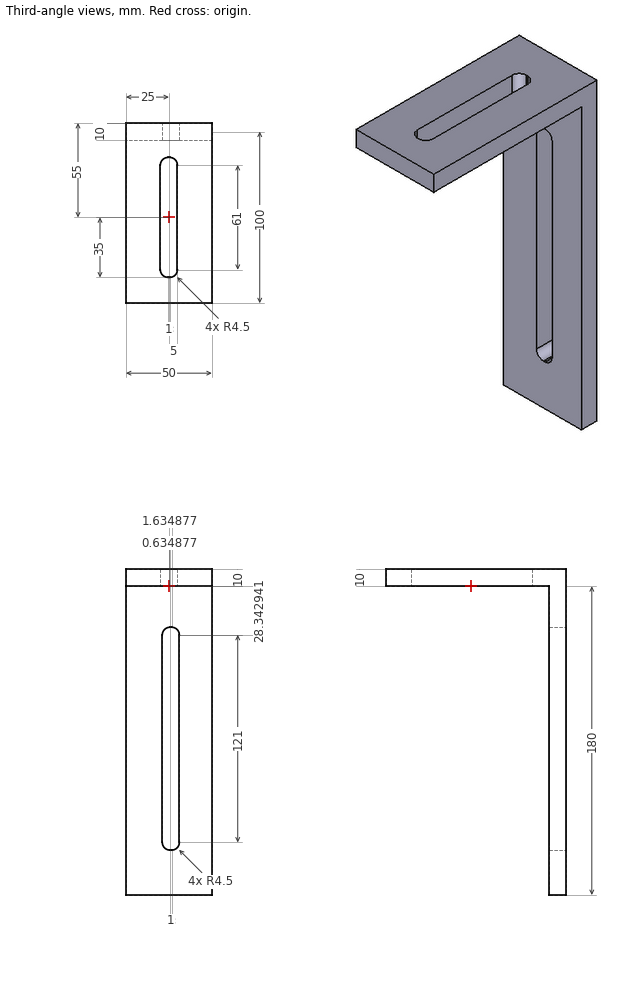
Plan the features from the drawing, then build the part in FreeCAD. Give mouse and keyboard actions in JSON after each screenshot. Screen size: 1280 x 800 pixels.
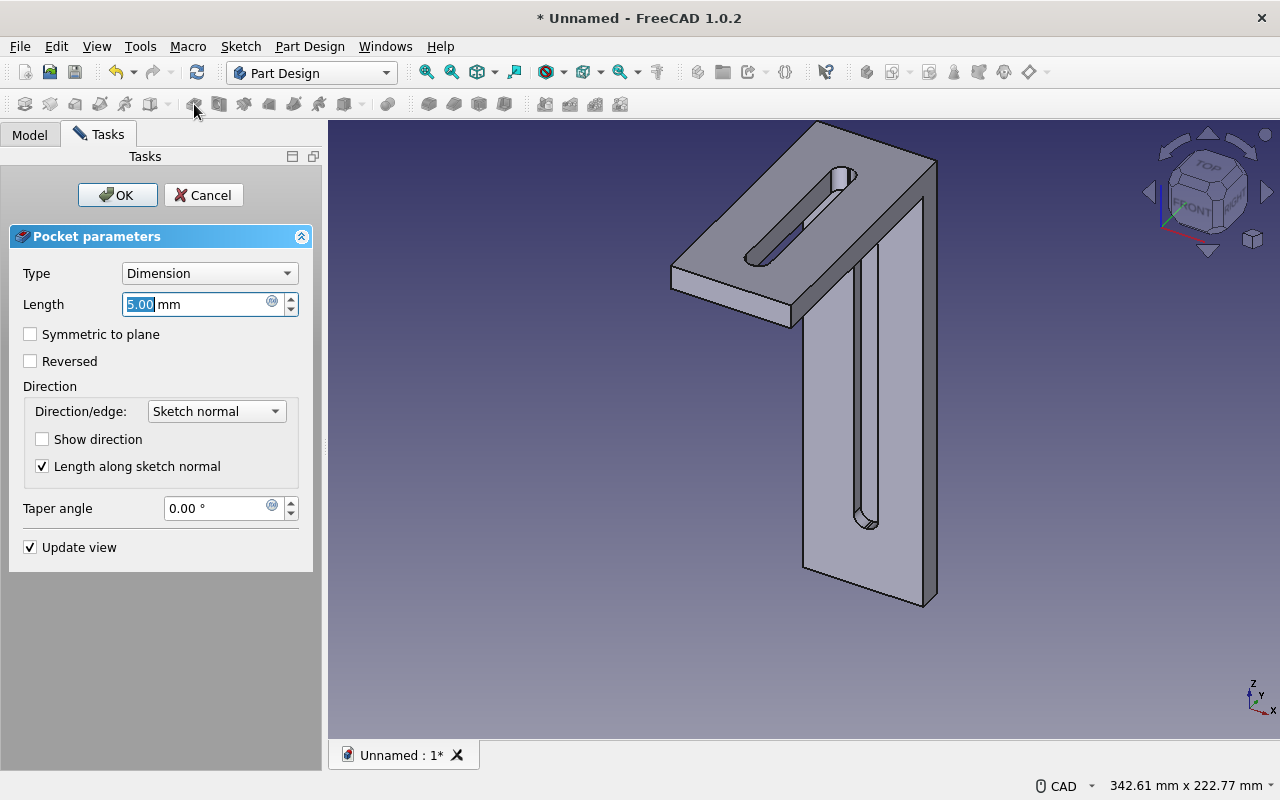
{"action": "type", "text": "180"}
{"action": "key", "text": "Tab"}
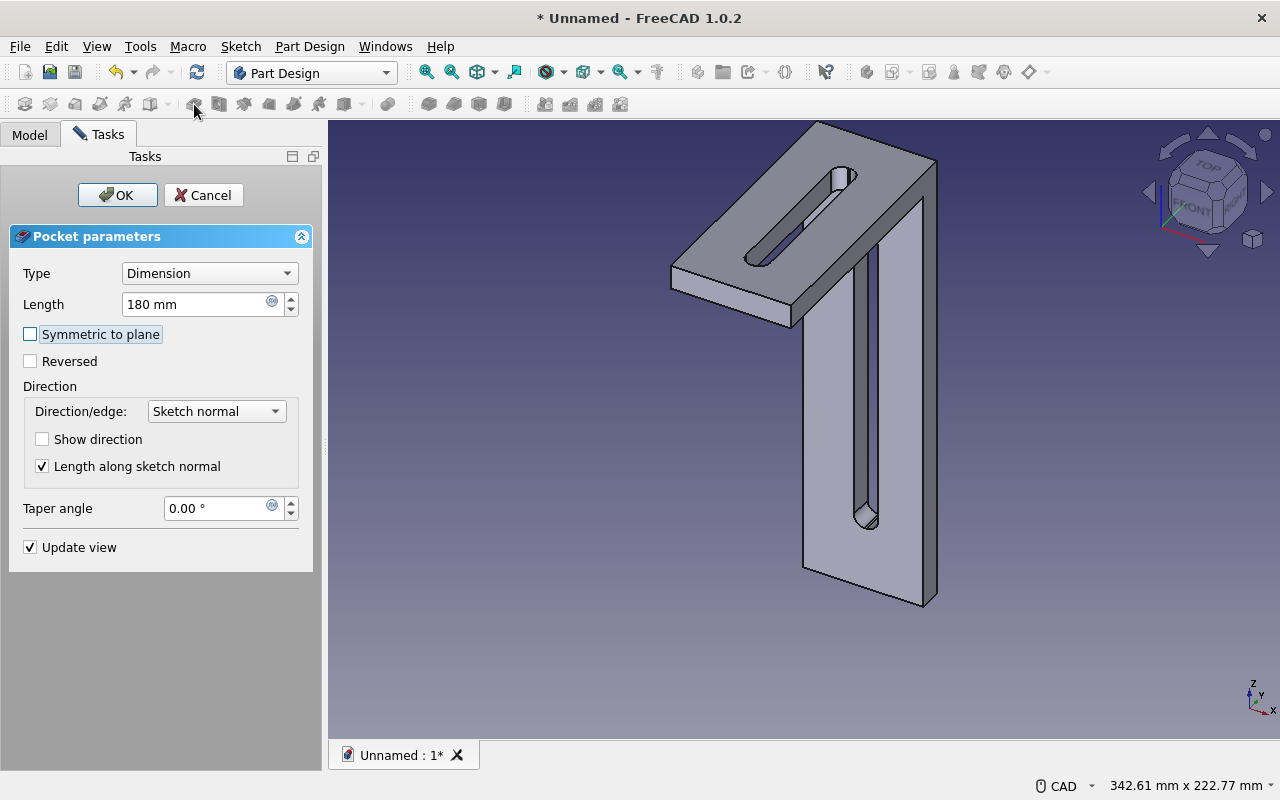
{"action": "left_click", "coordinate": [118, 195]}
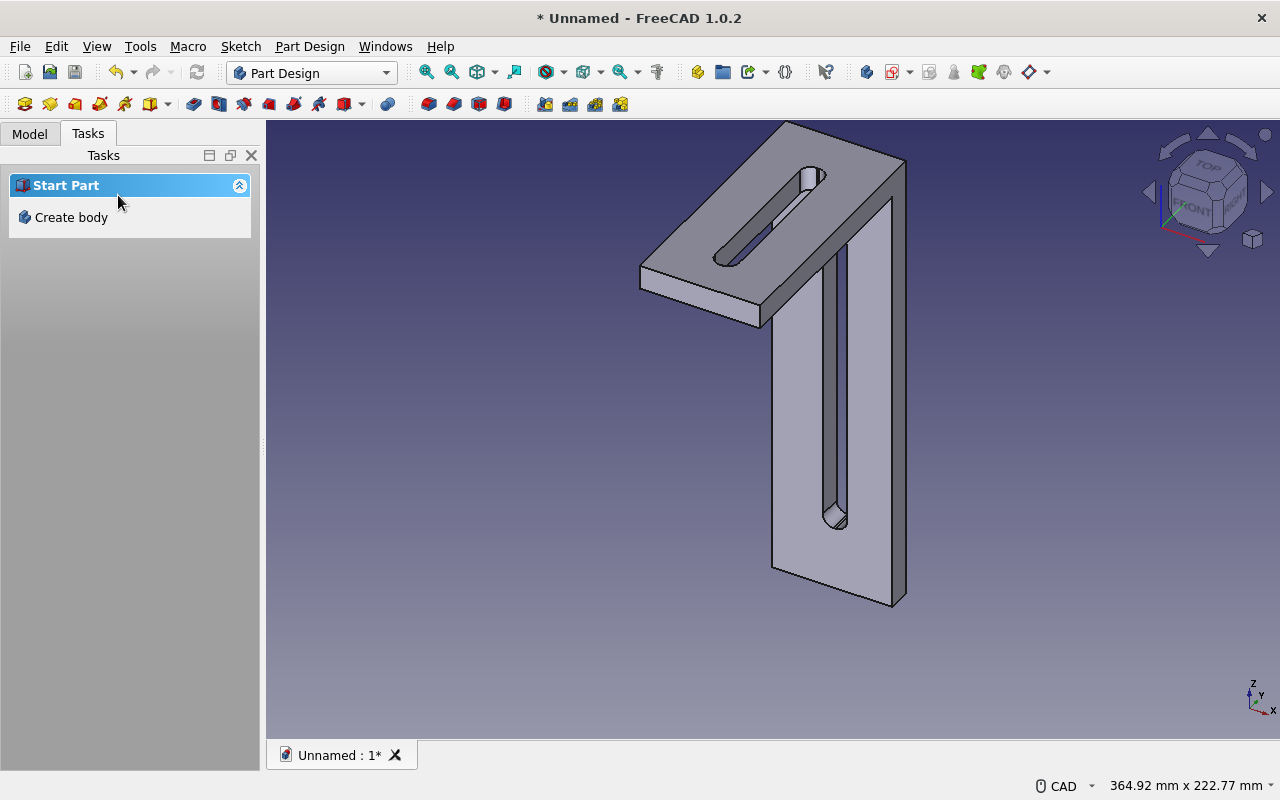
{"action": "key", "text": "0"}